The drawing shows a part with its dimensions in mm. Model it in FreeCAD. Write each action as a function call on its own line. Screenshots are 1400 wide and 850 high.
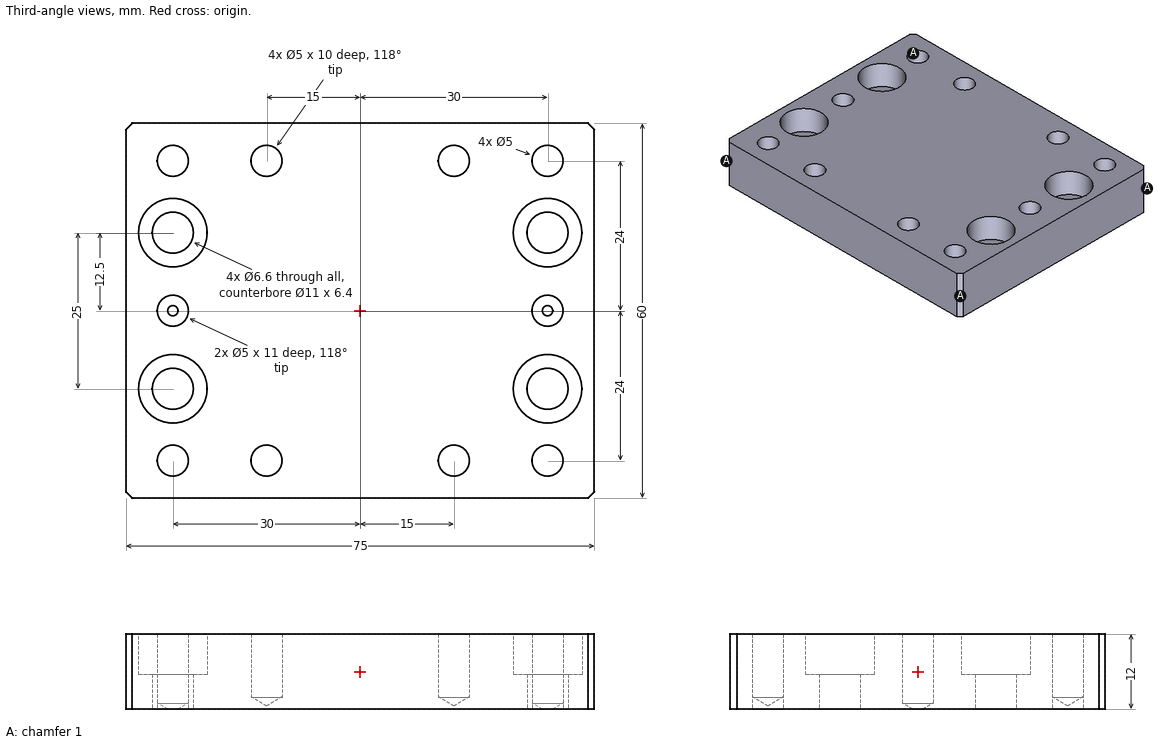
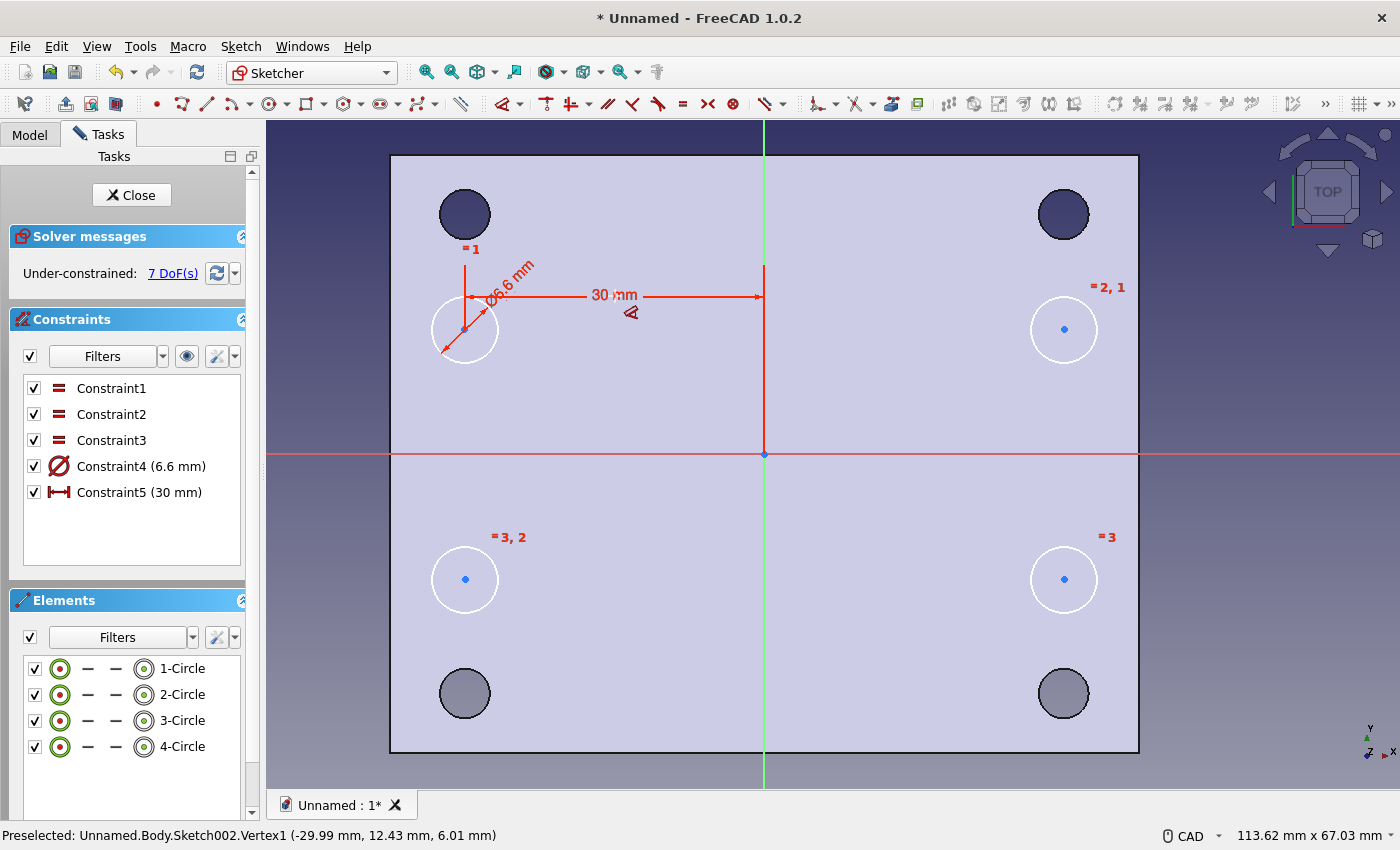
click(1064, 330)
click(914, 296)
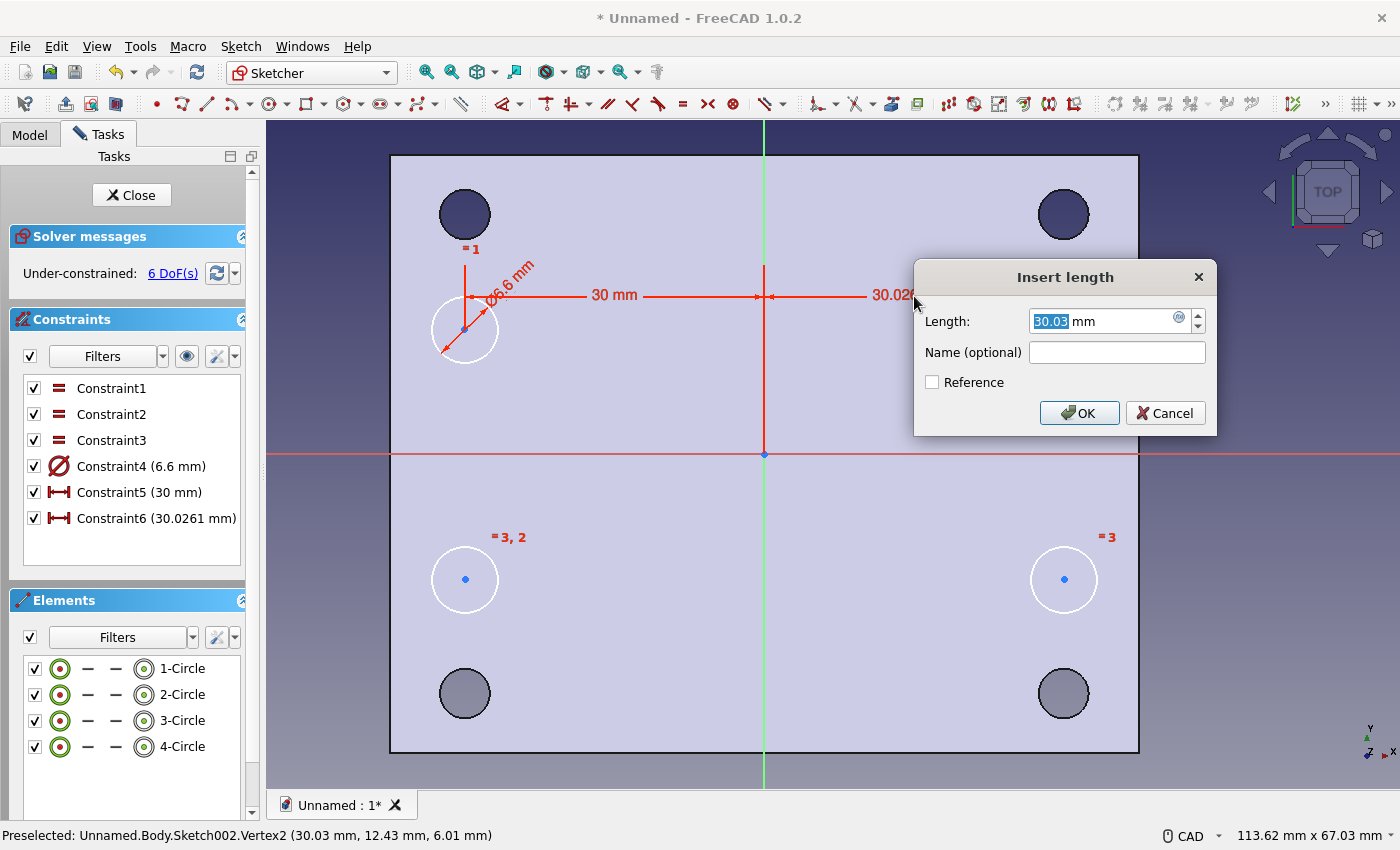
text(30)
key(Return)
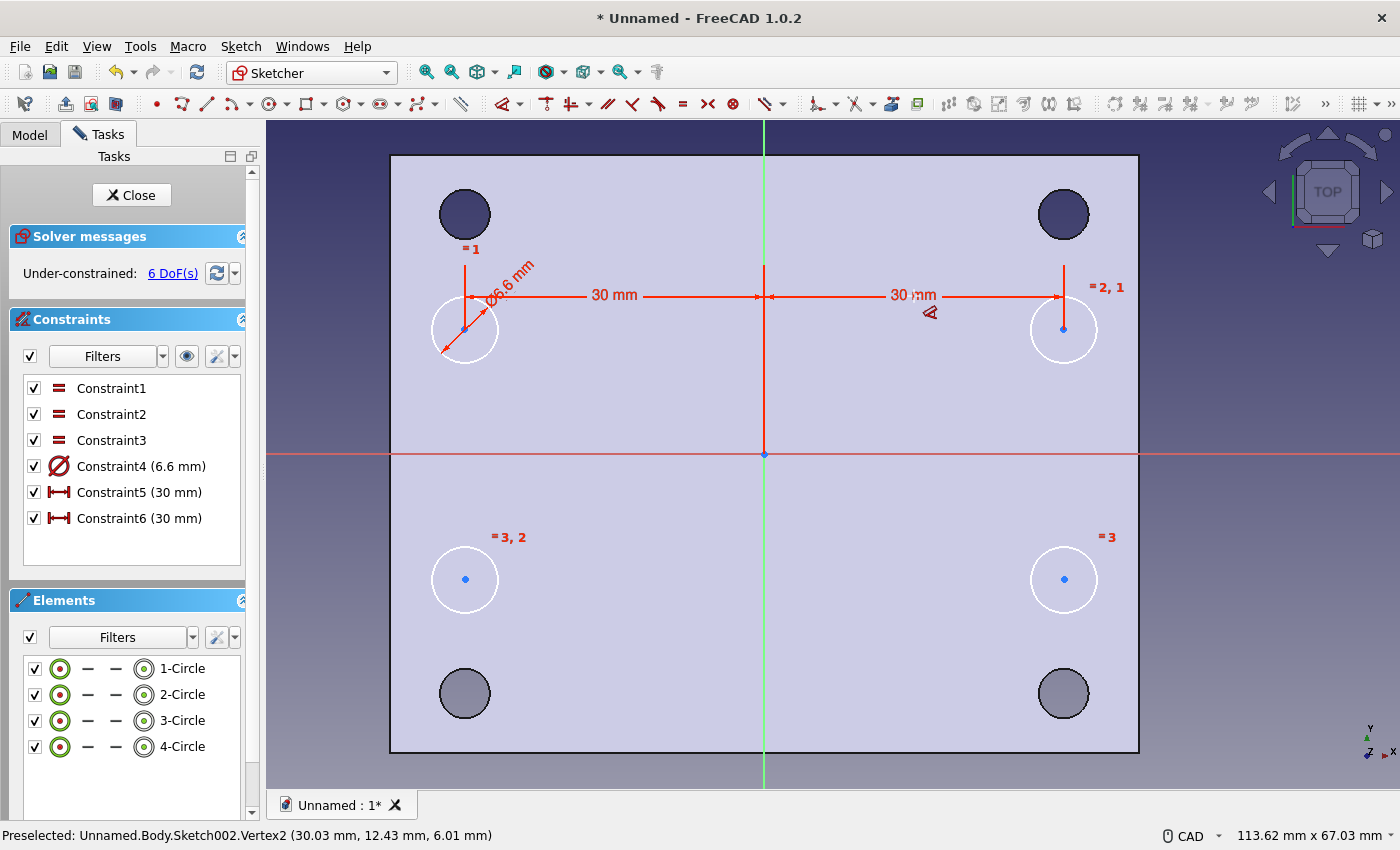
click(465, 580)
click(615, 614)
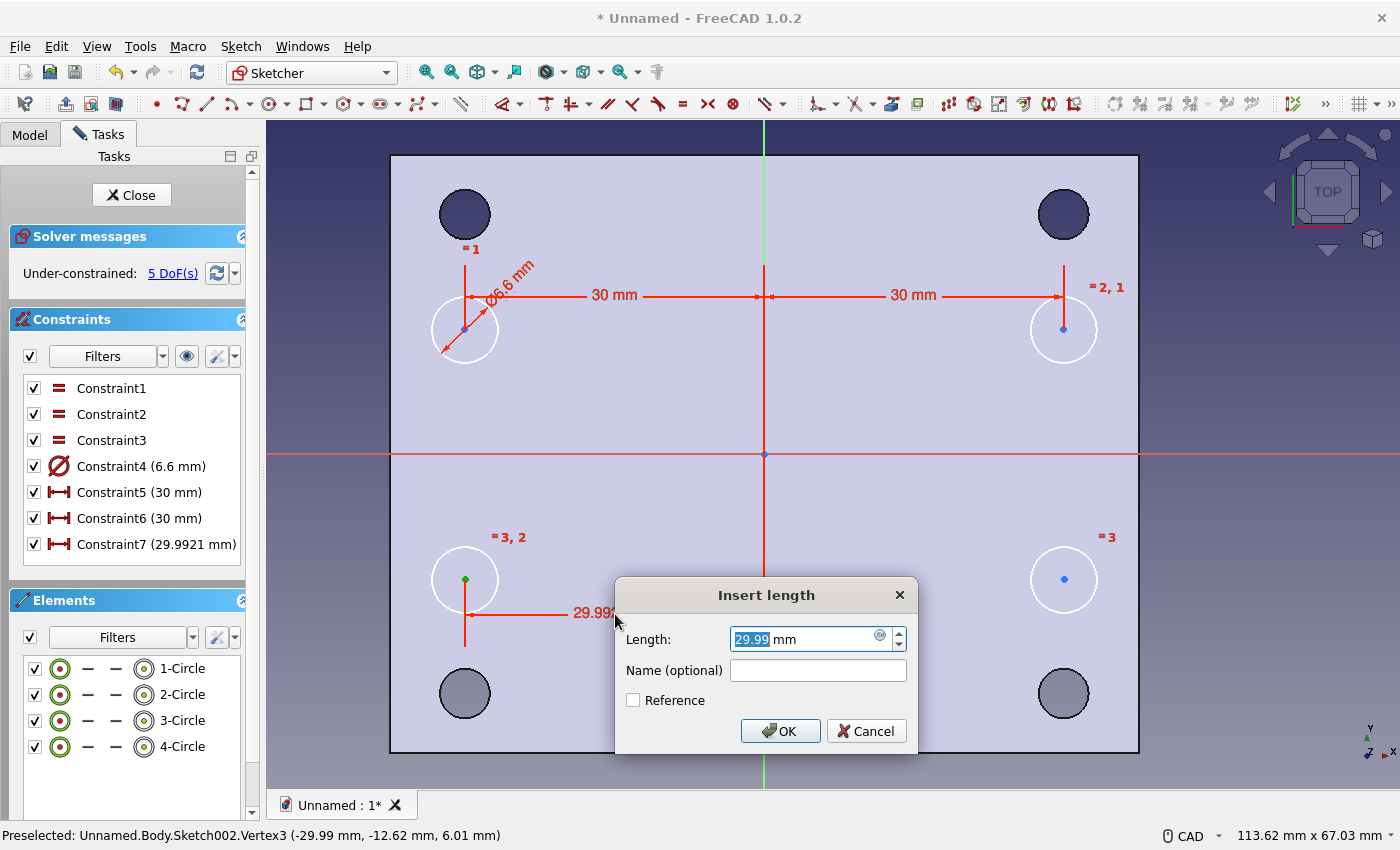
text(30)
key(Return)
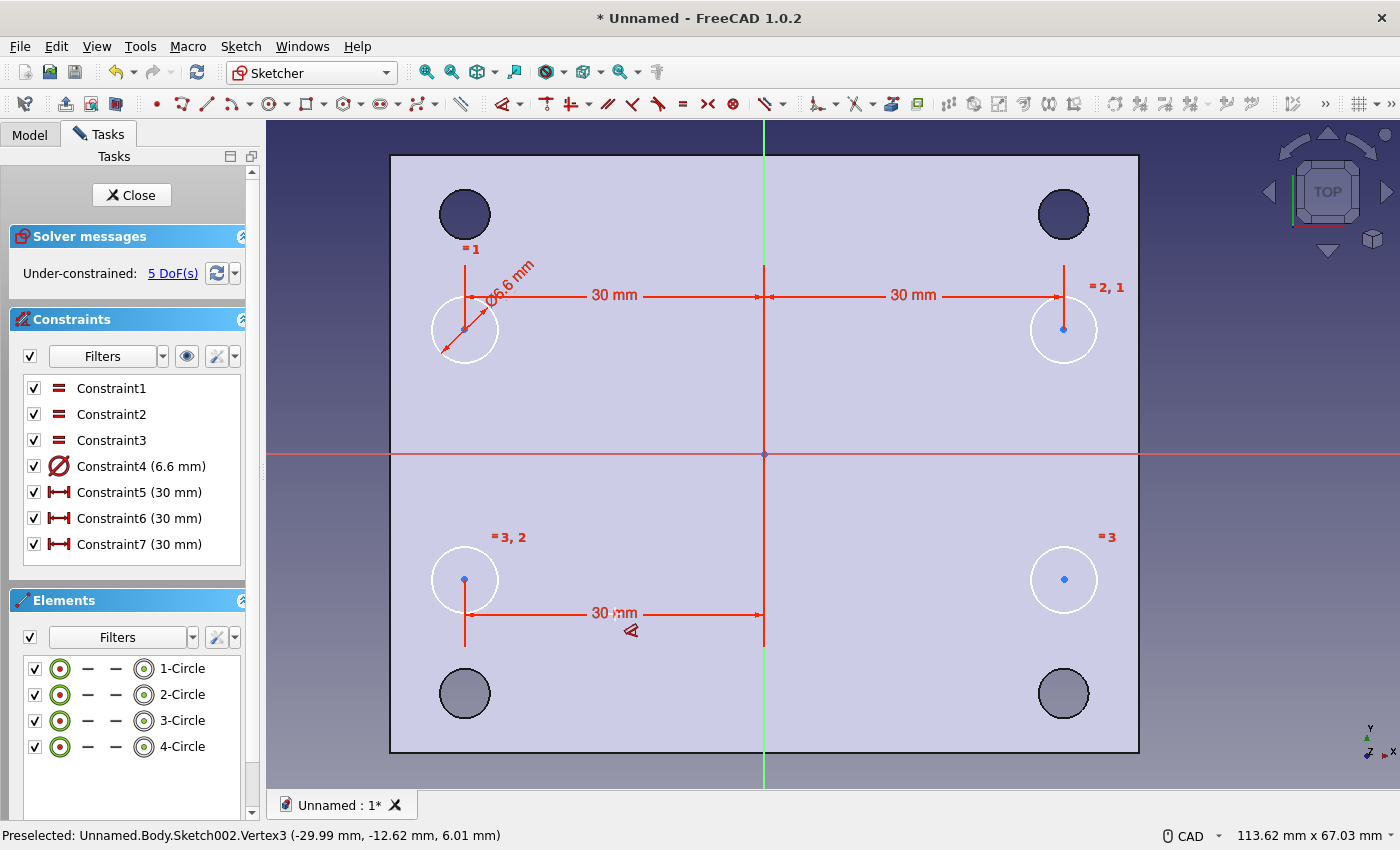
click(1064, 580)
click(914, 614)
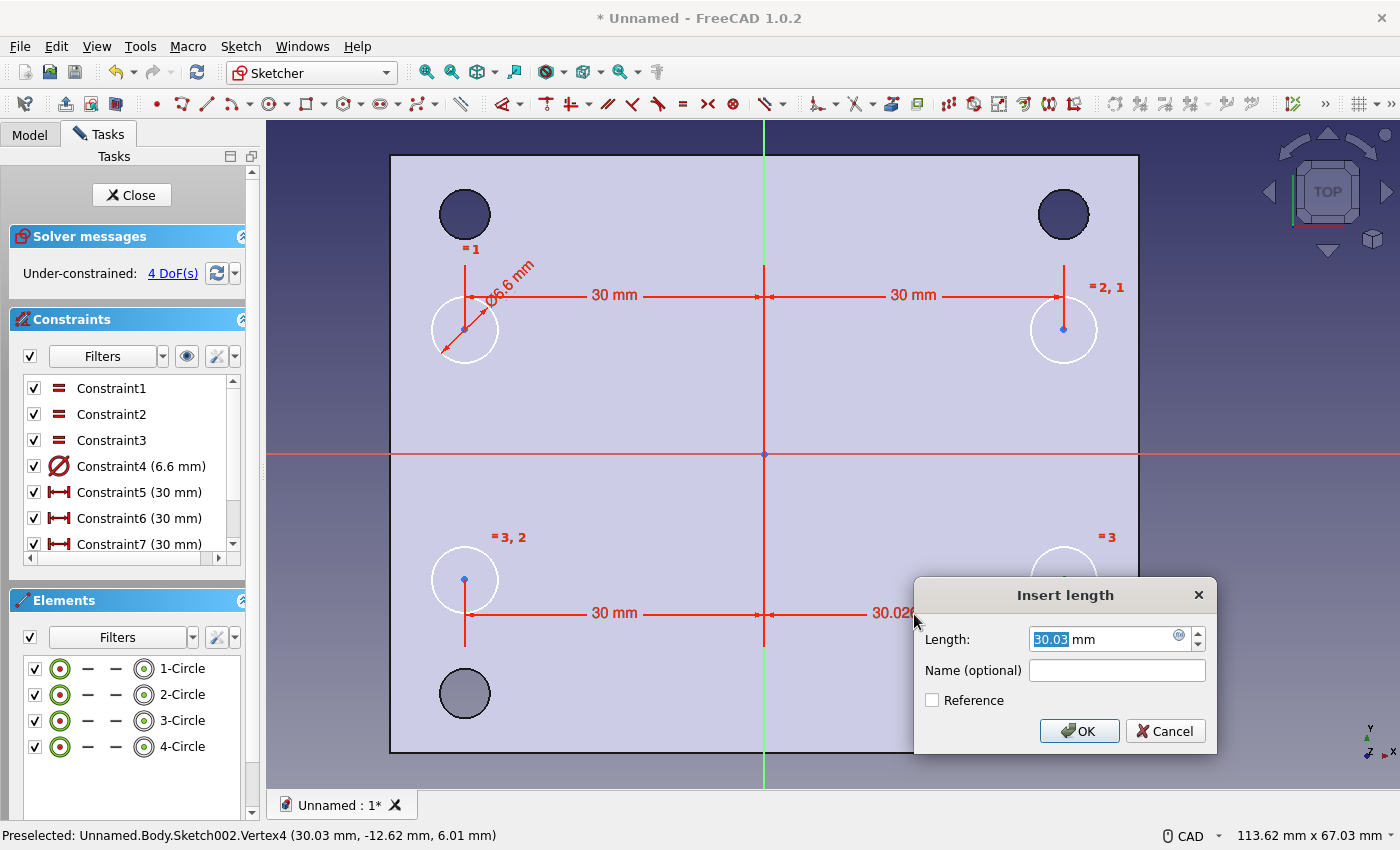
text(30)
key(Return)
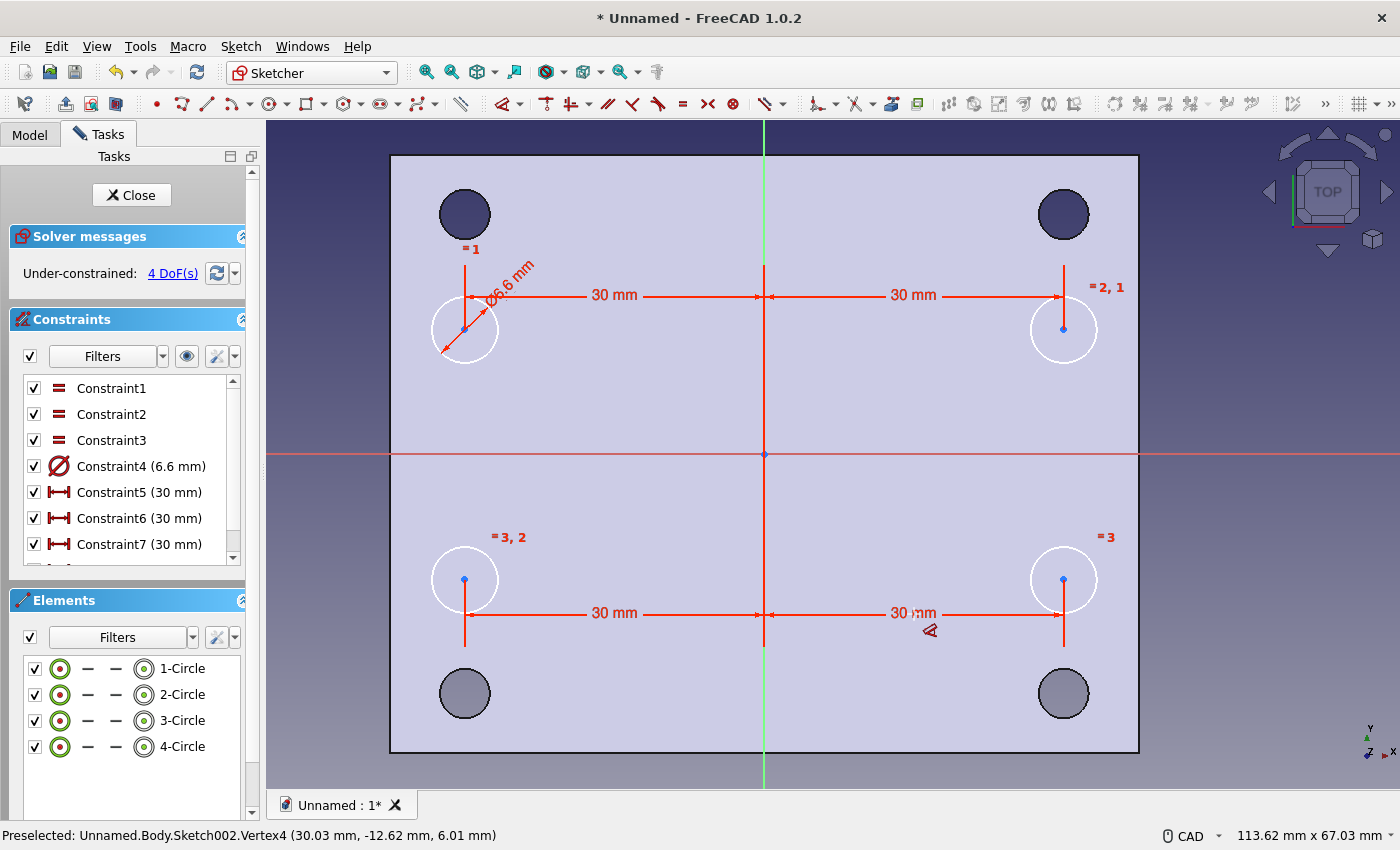
click(465, 330)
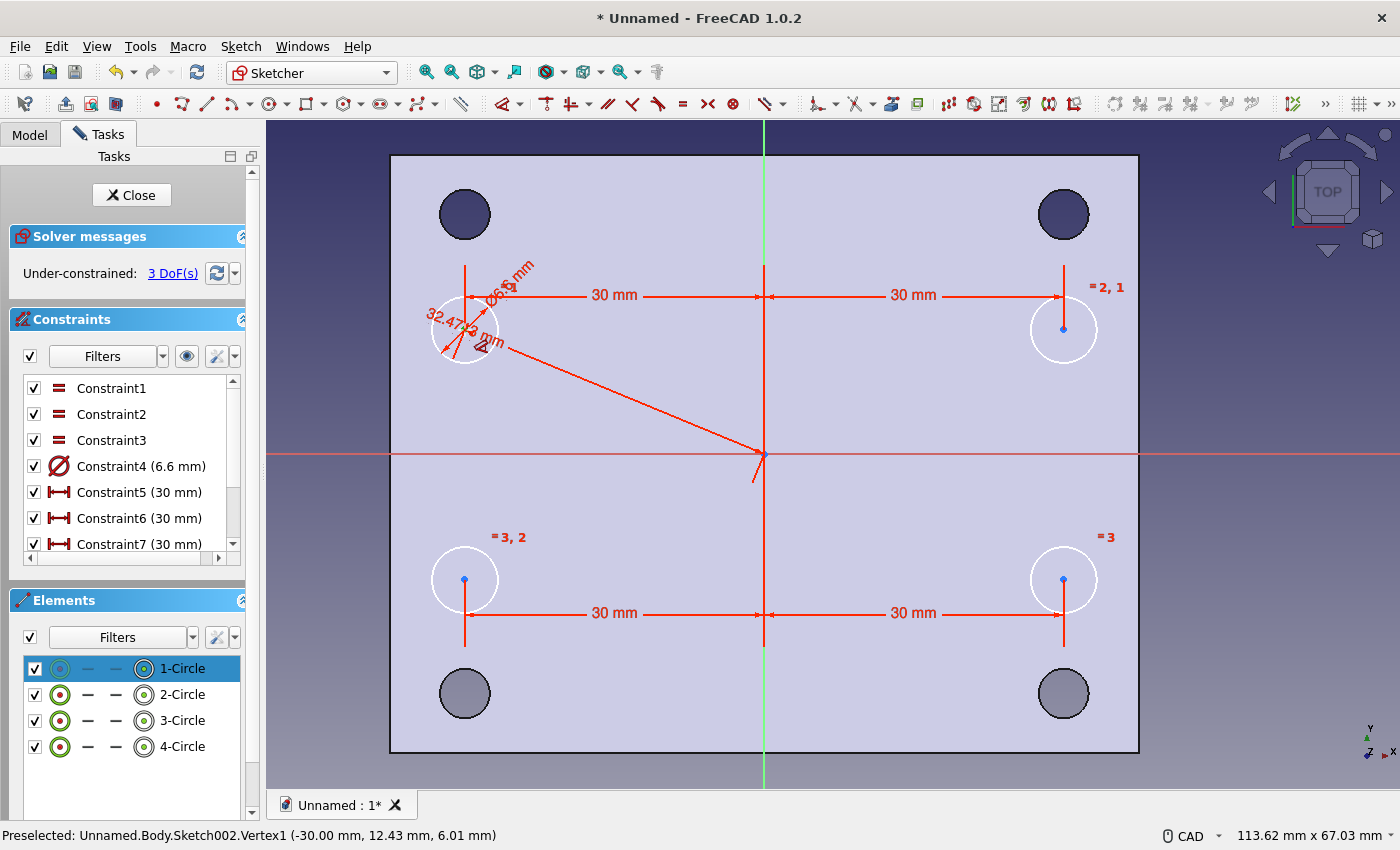
click(465, 580)
click(431, 398)